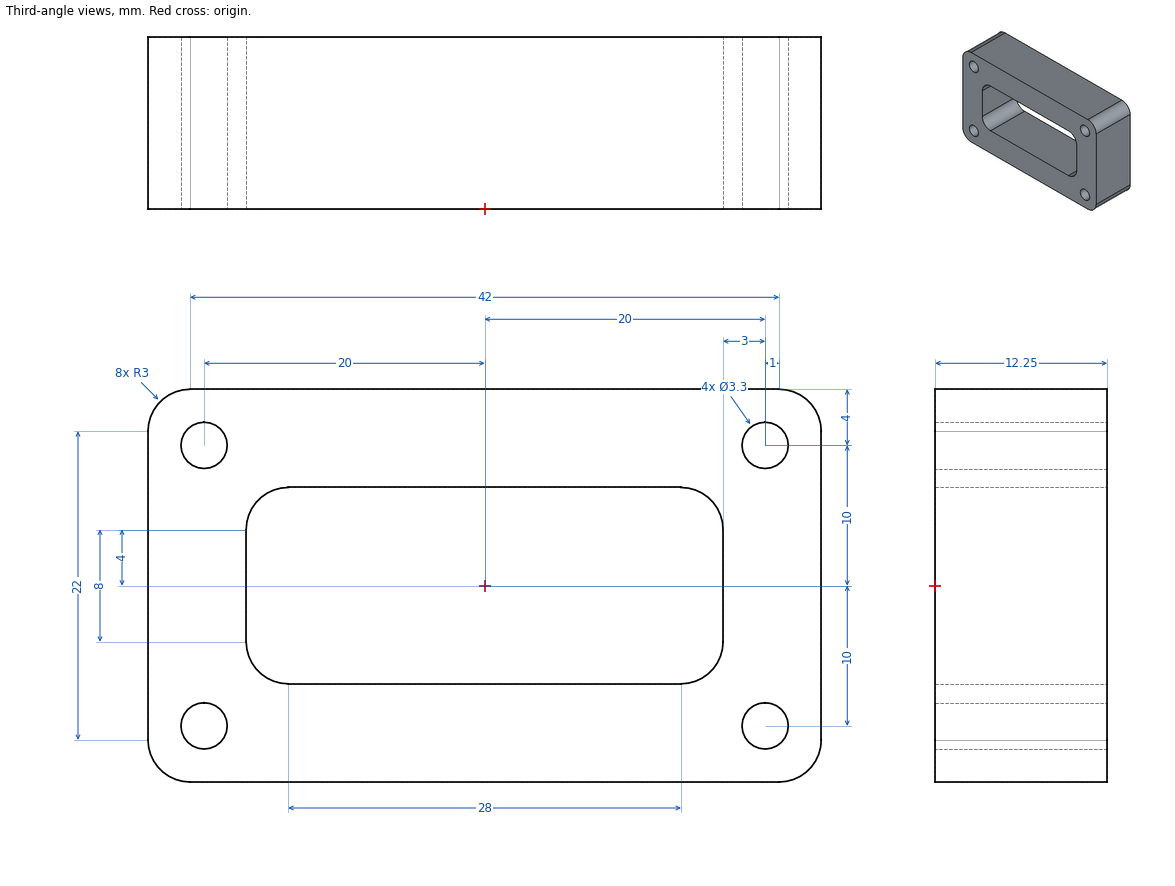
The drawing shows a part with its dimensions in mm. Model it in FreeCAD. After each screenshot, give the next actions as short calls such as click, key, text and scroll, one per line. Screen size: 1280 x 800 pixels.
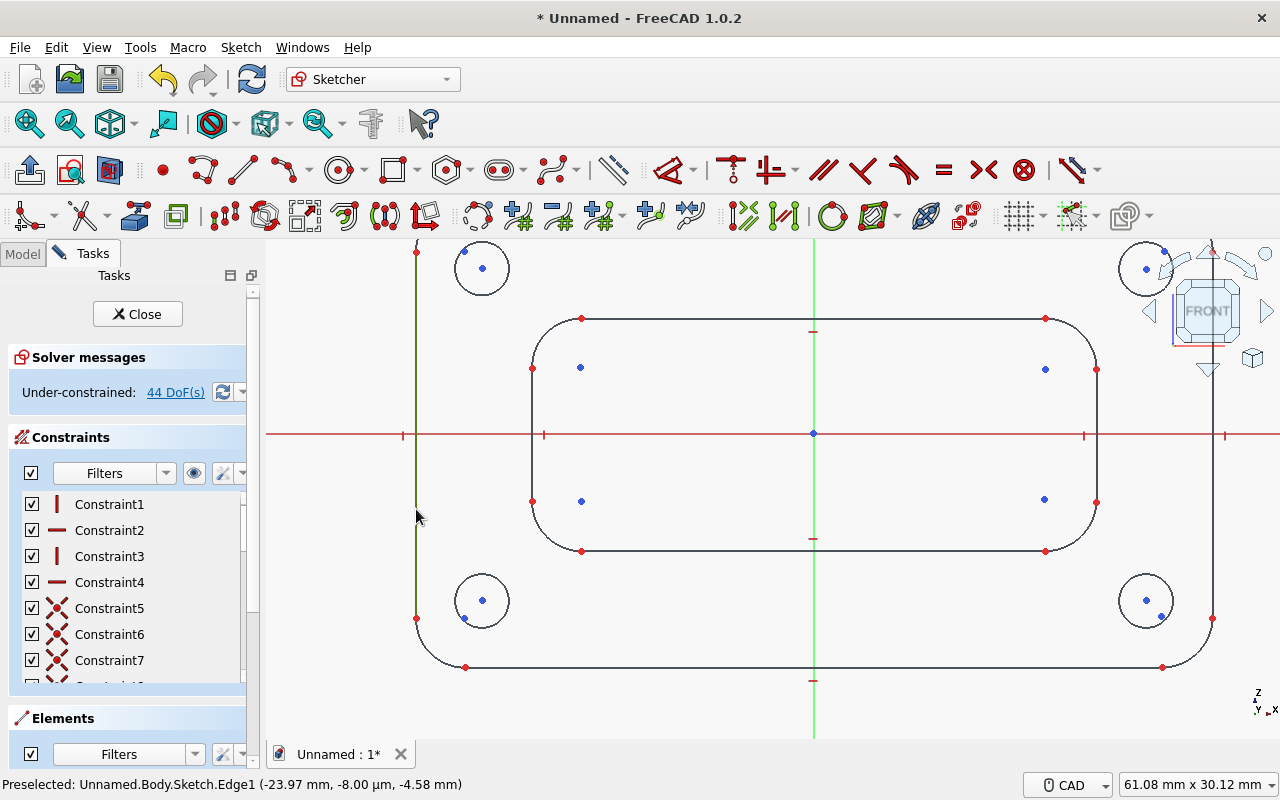
scroll(482, 601, down, 2)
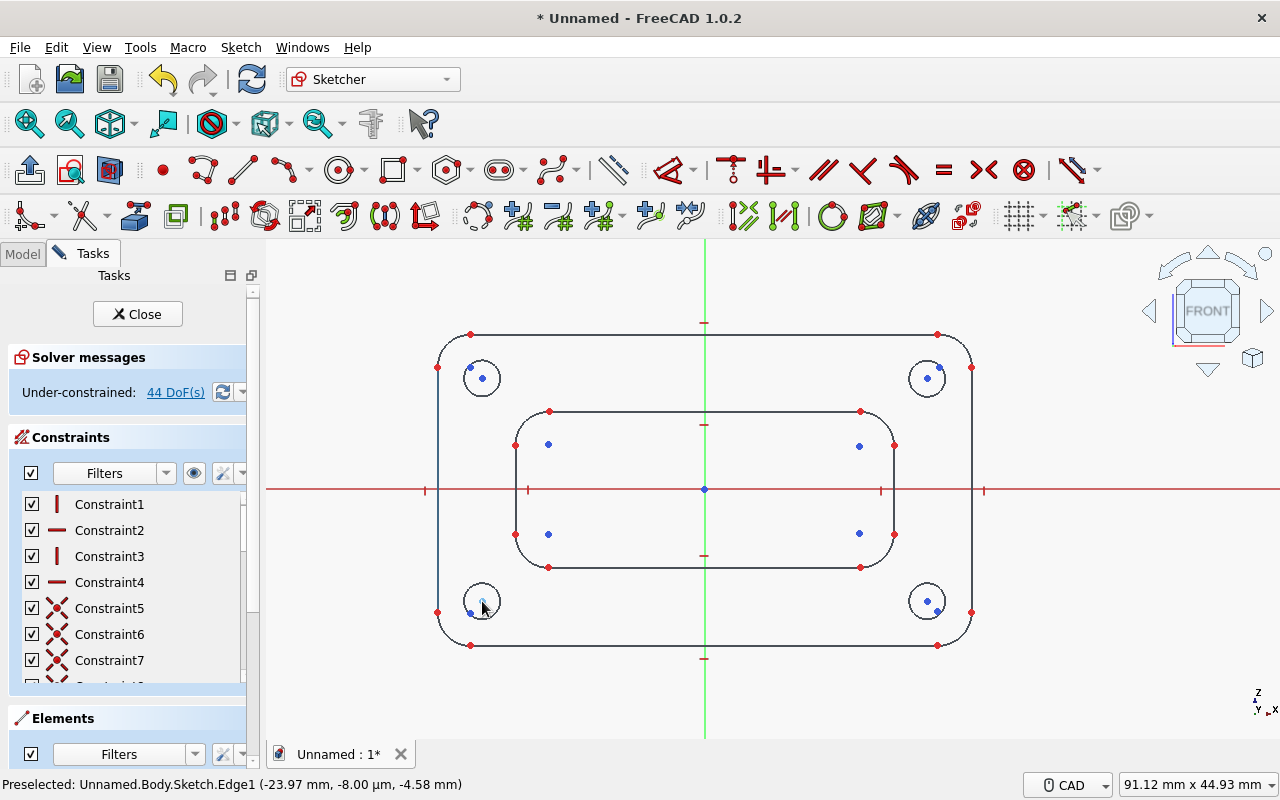
click(456, 338)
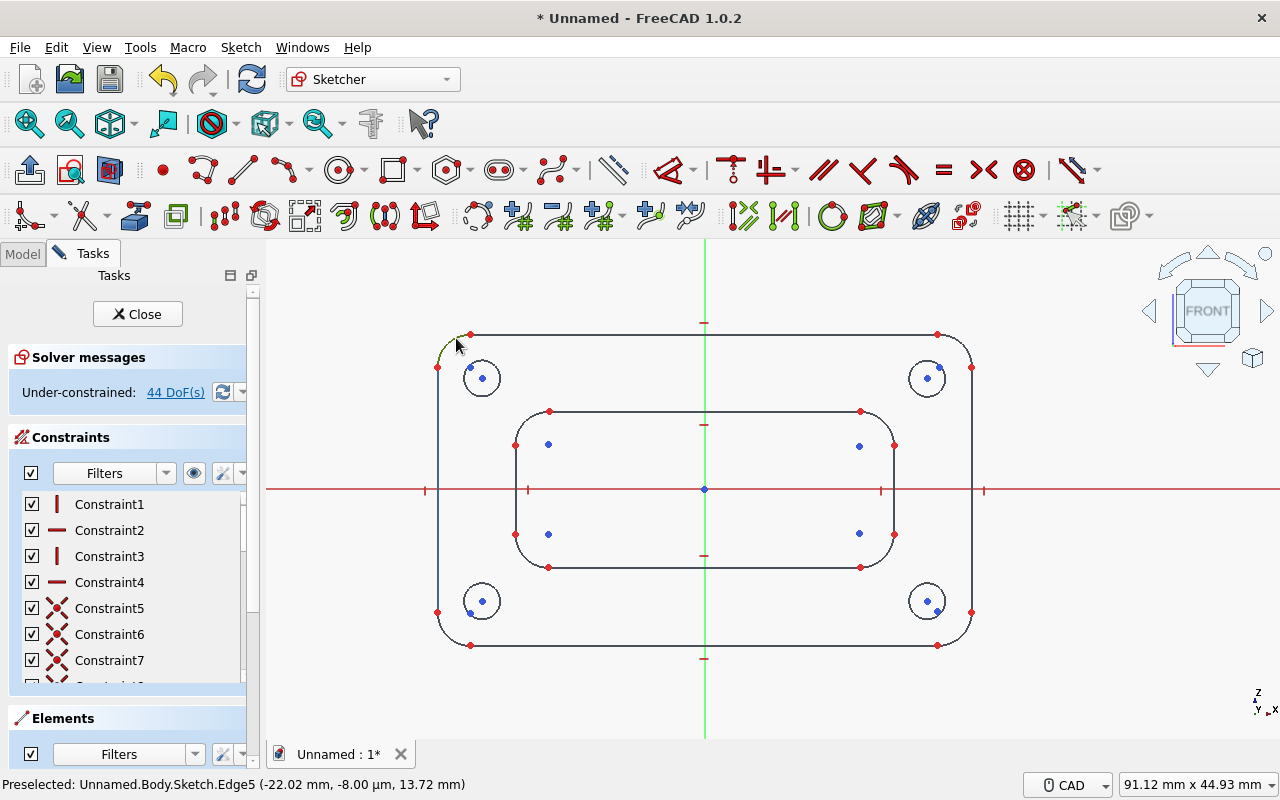
click(904, 170)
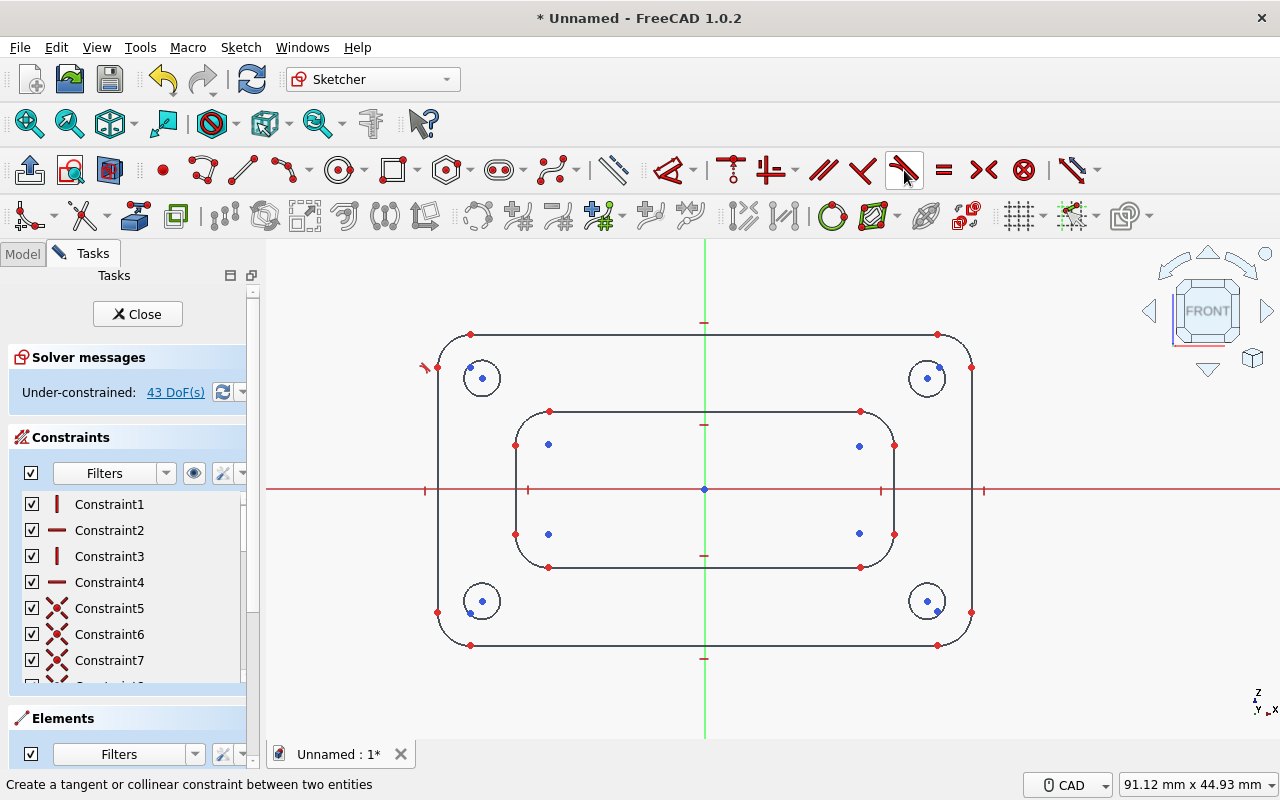
click(438, 539)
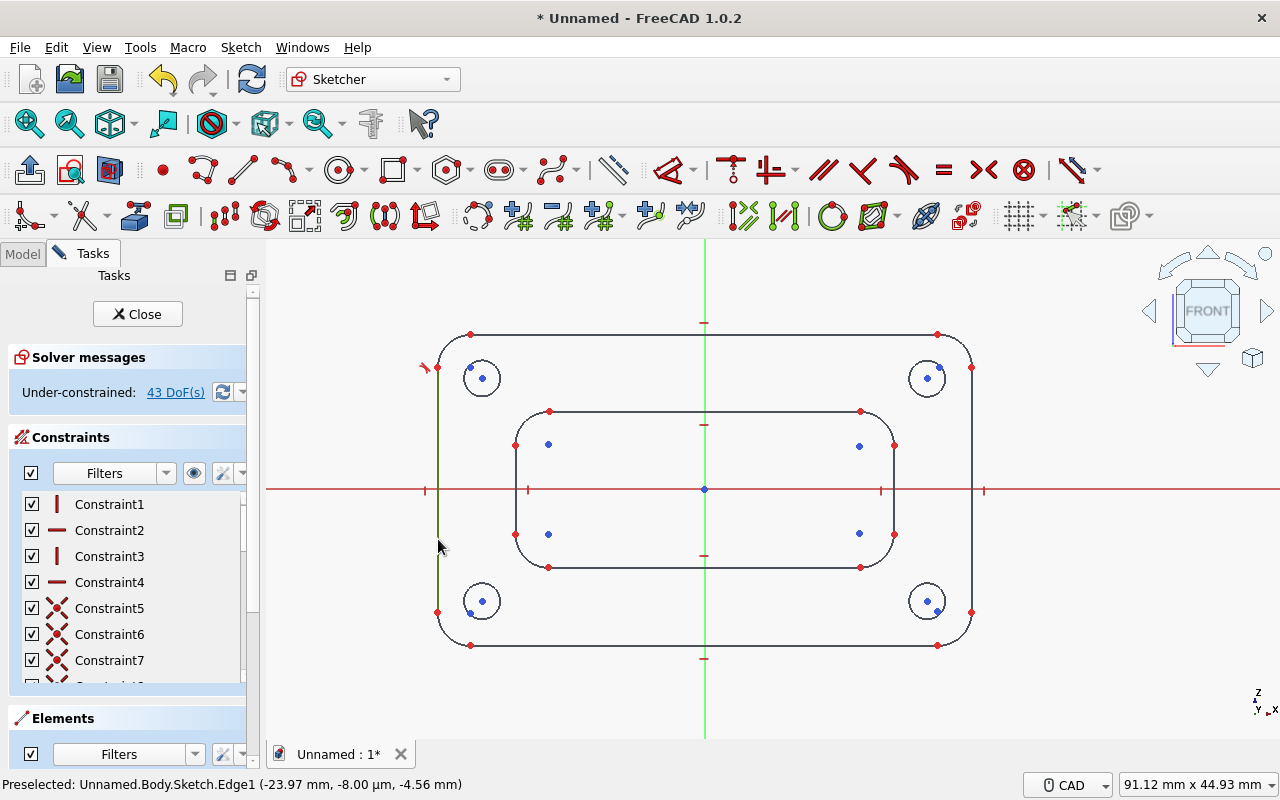
click(441, 628)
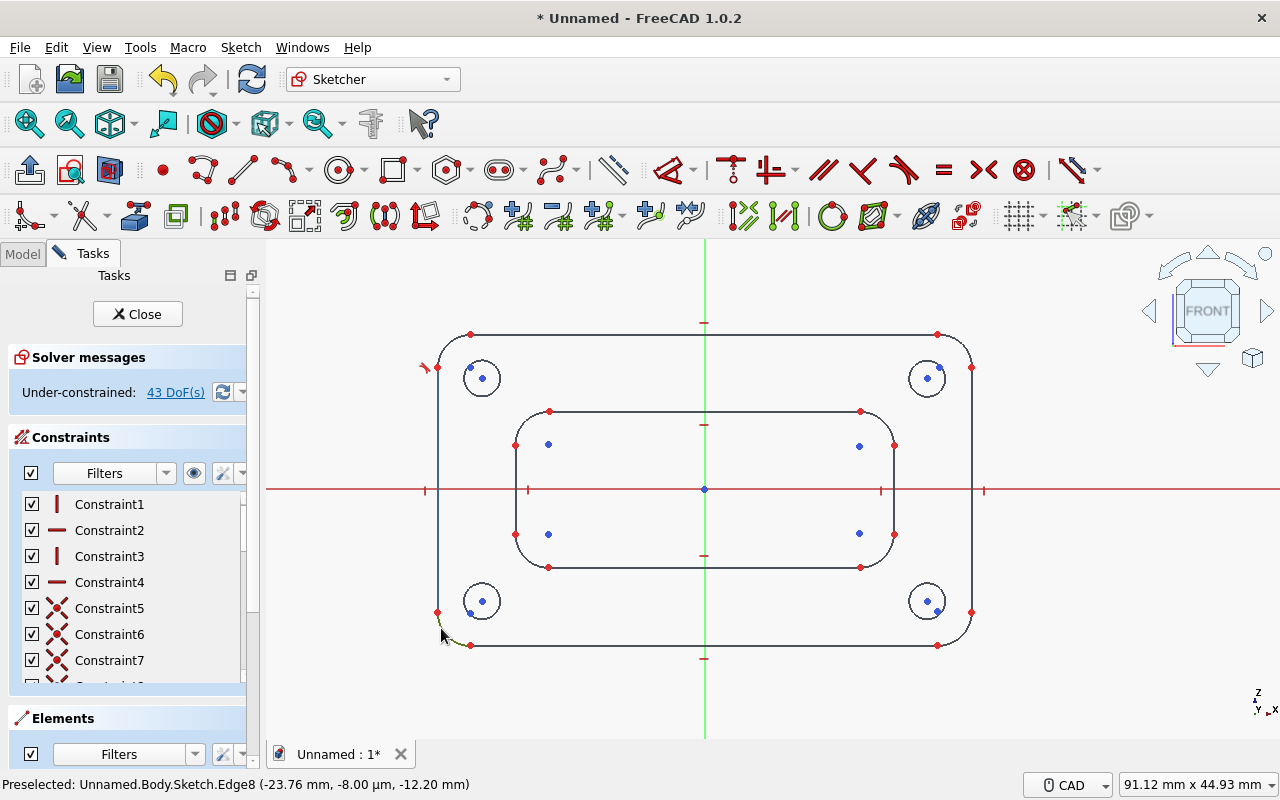
click(904, 170)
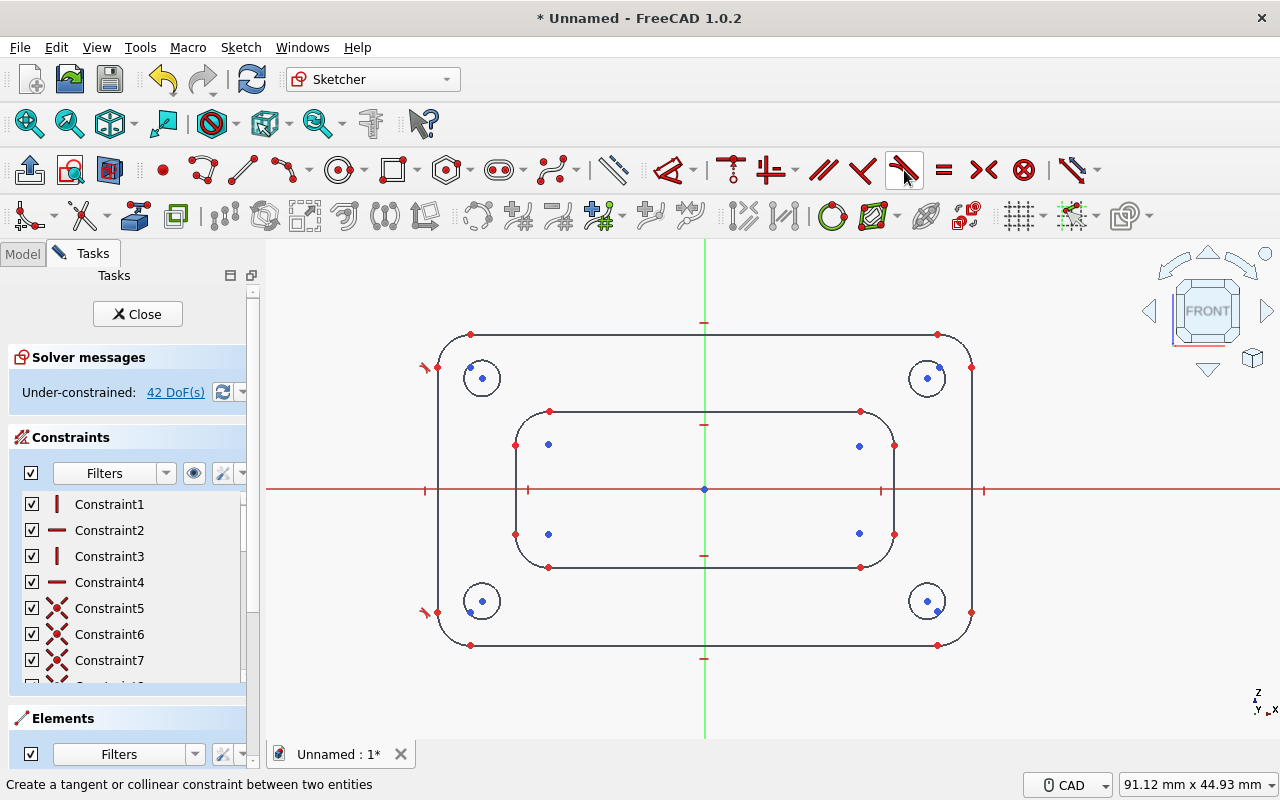
click(611, 335)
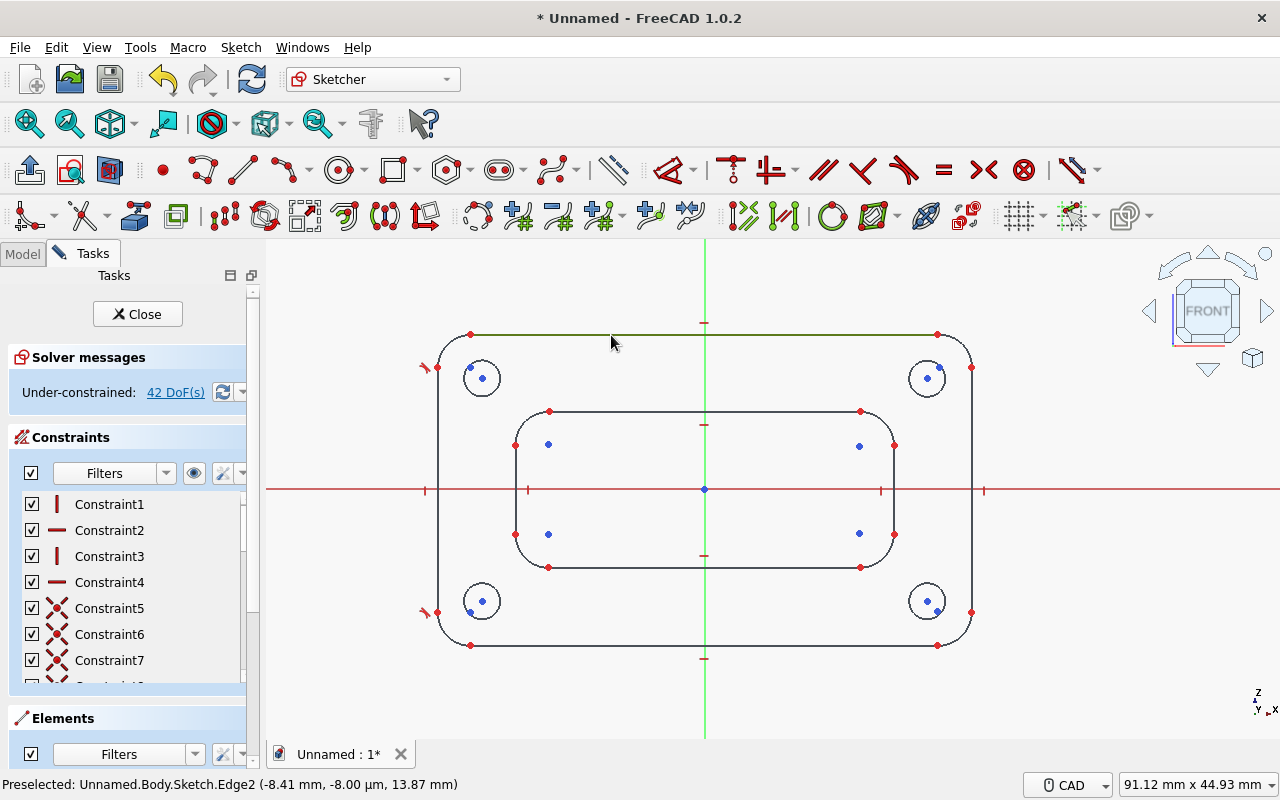
click(456, 338)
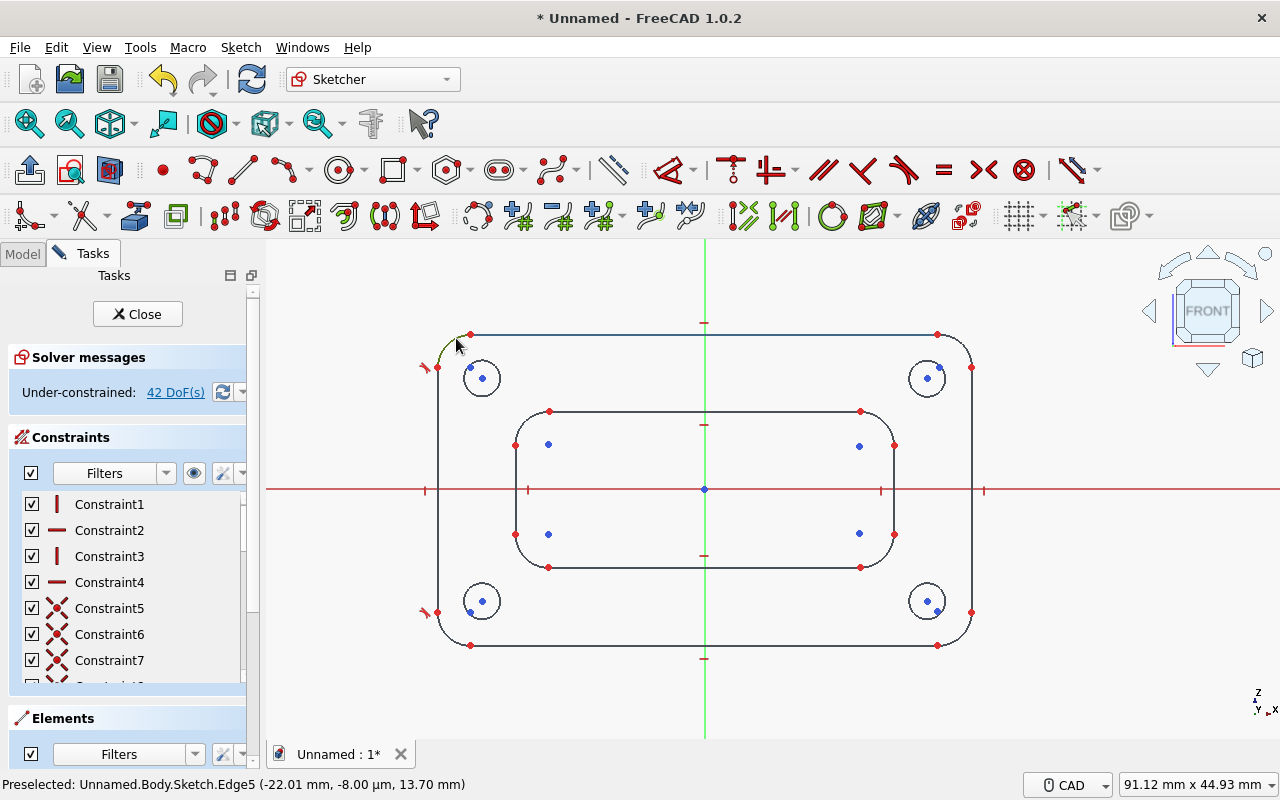
click(904, 170)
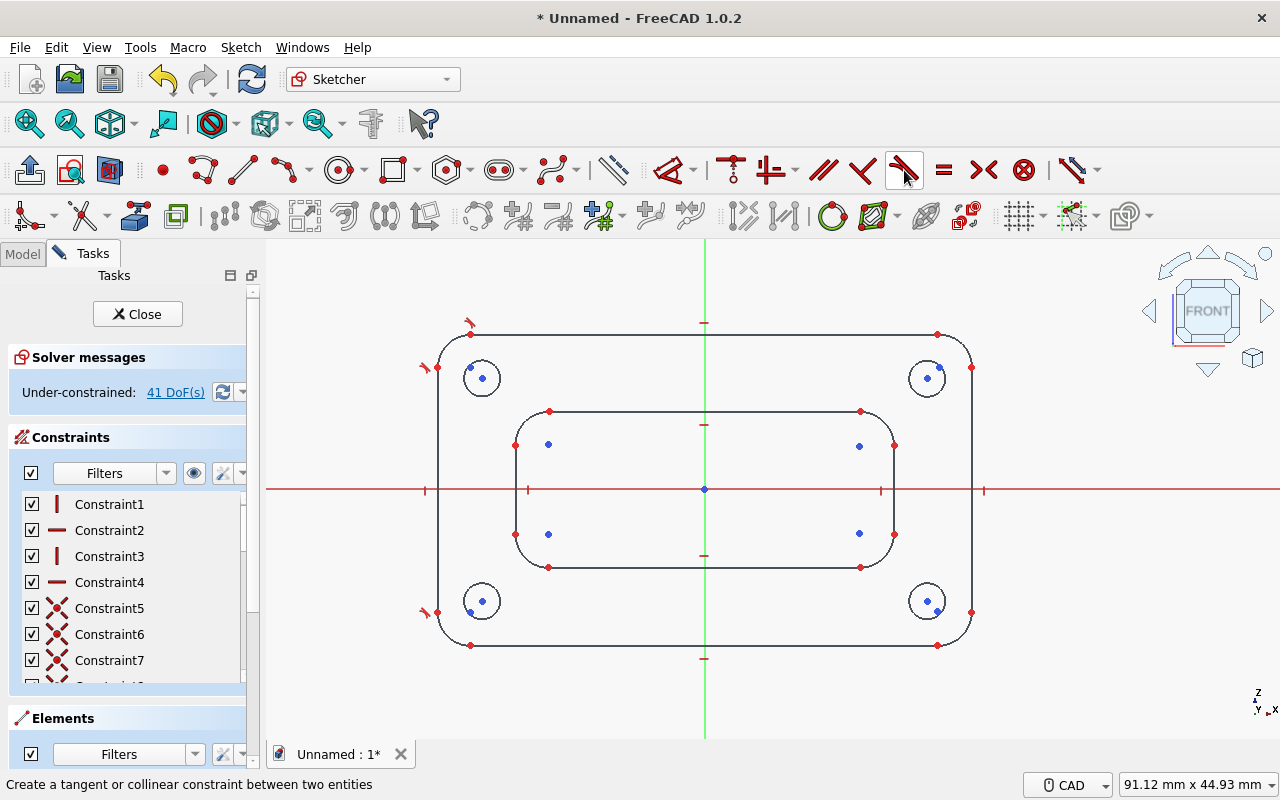
click(611, 335)